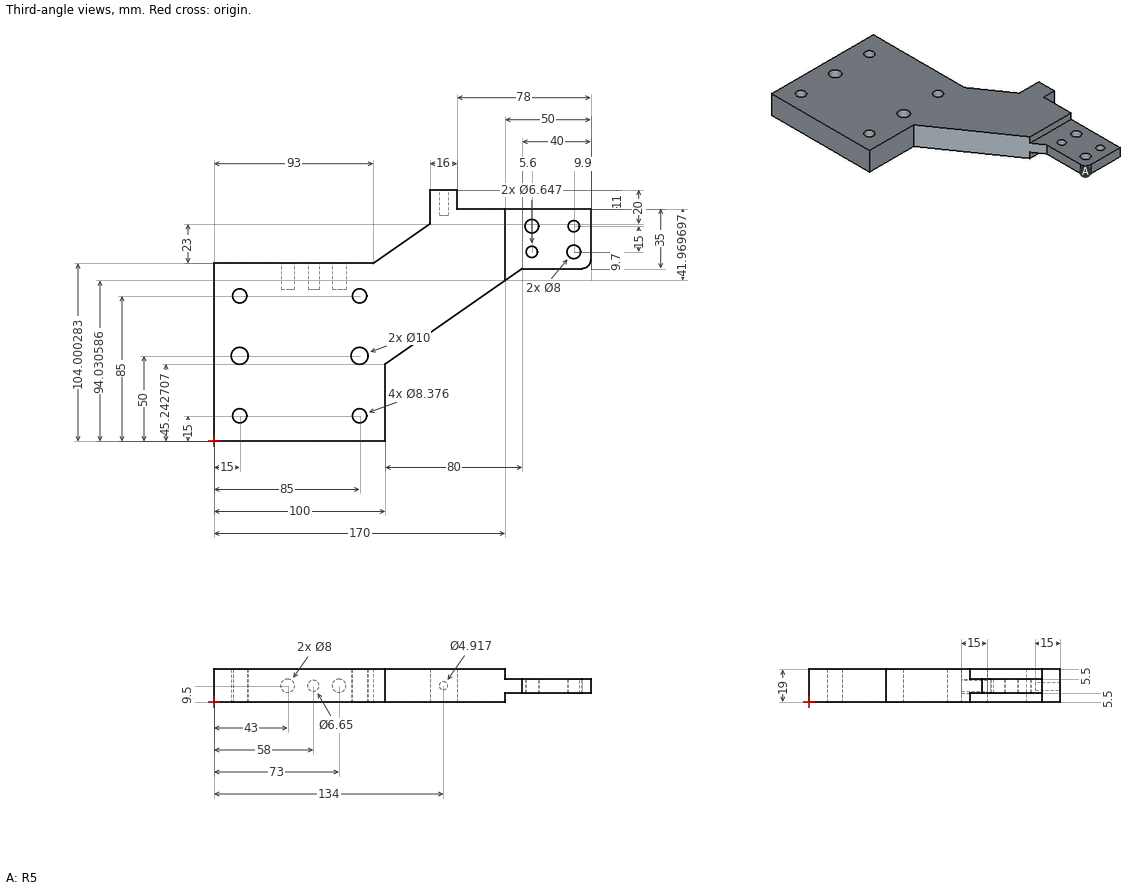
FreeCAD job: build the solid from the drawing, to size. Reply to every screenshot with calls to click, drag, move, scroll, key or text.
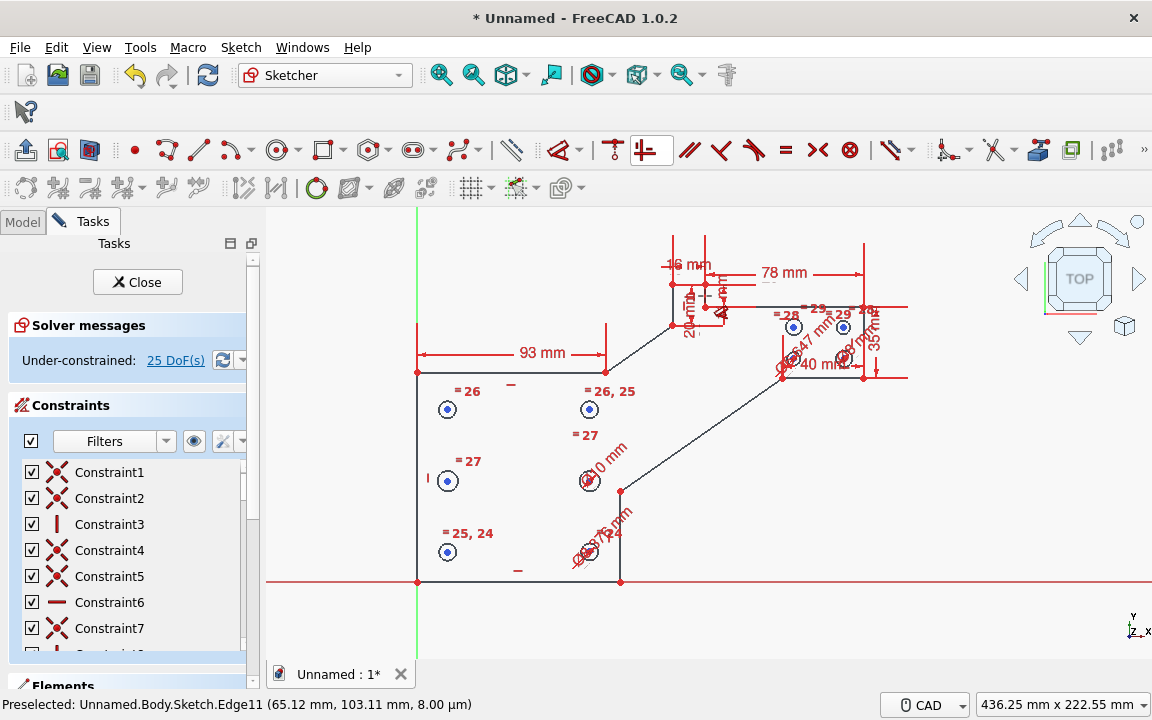
click(590, 552)
click(503, 616)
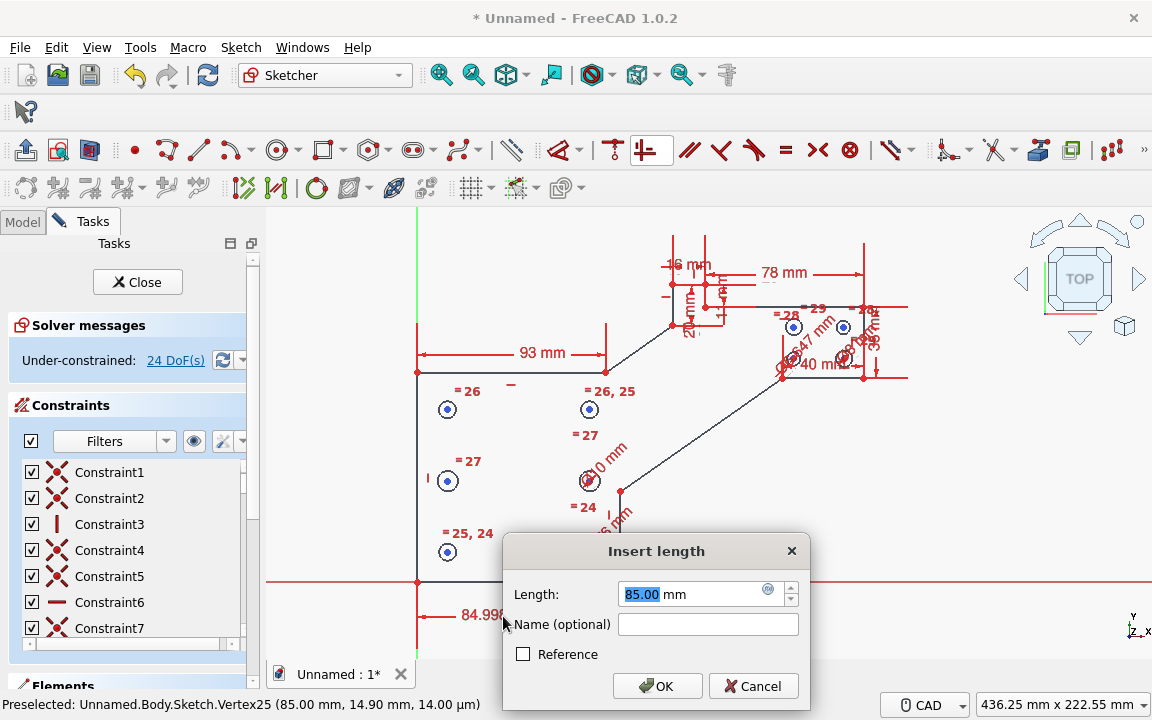
text(85)
key(Return)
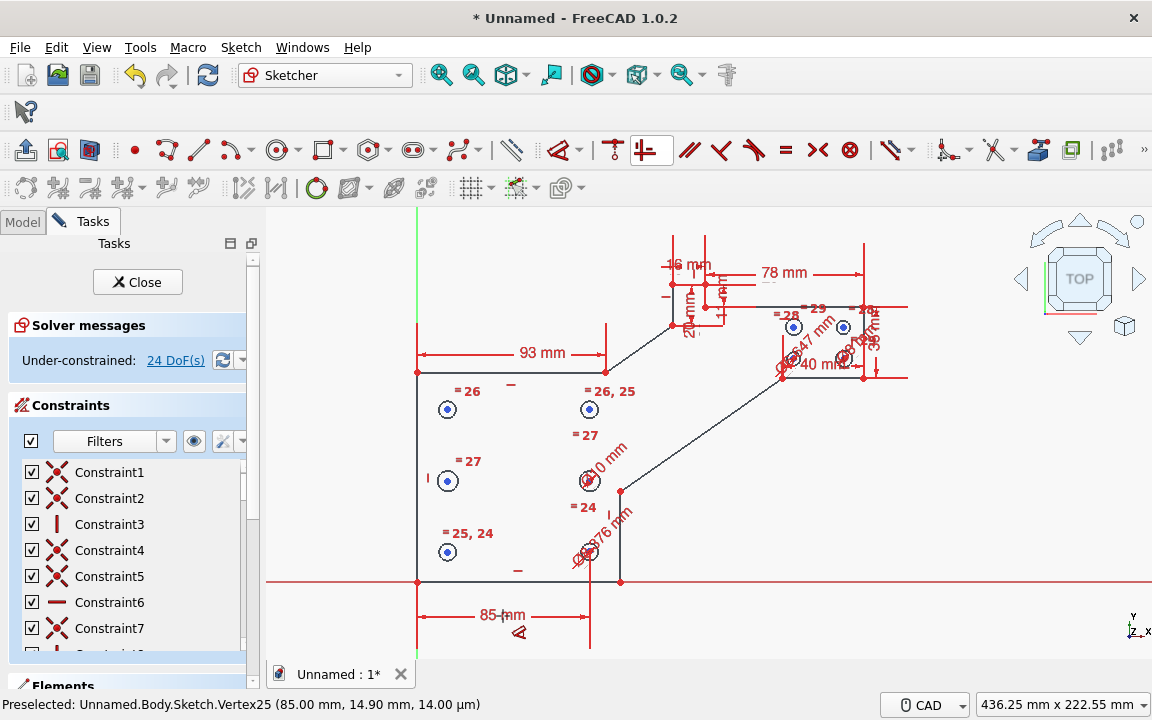
scroll(590, 552, up, 2)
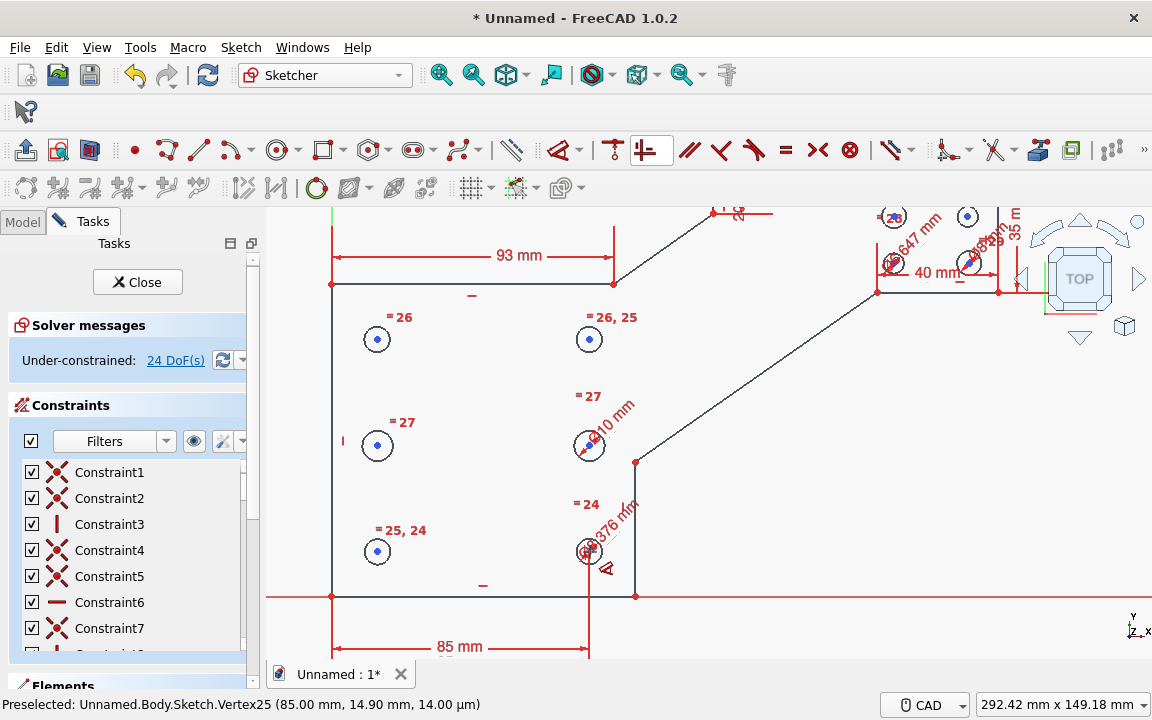
click(589, 552)
click(298, 574)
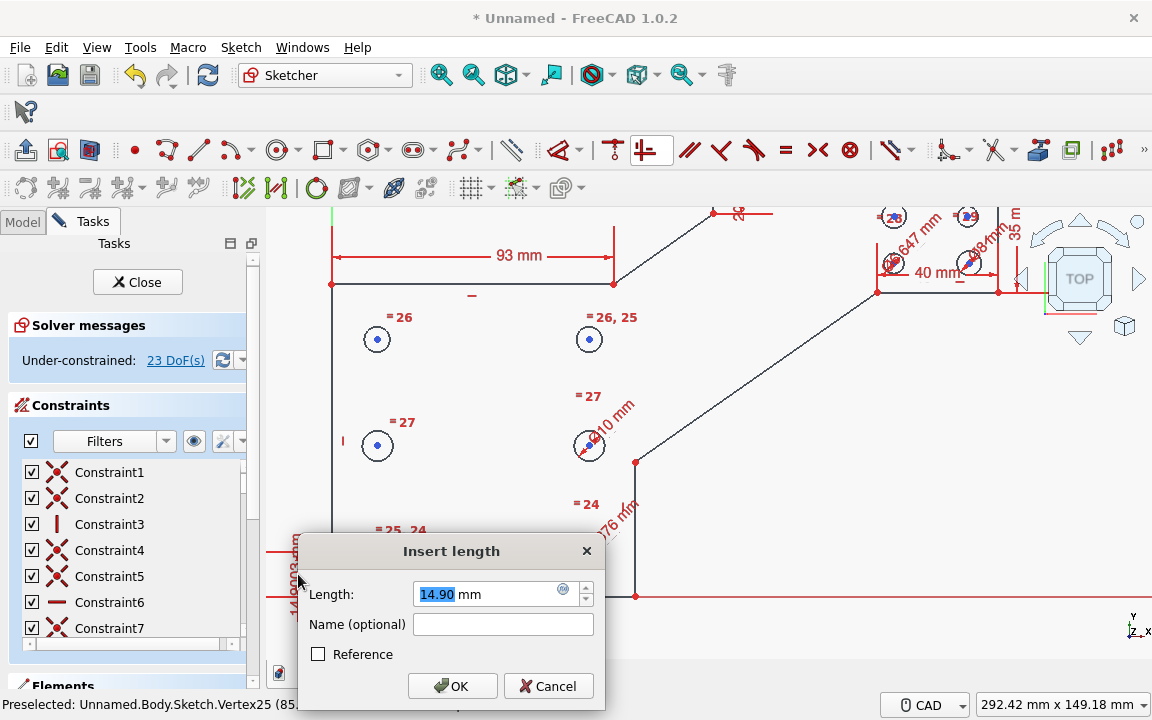
text(15)
key(Return)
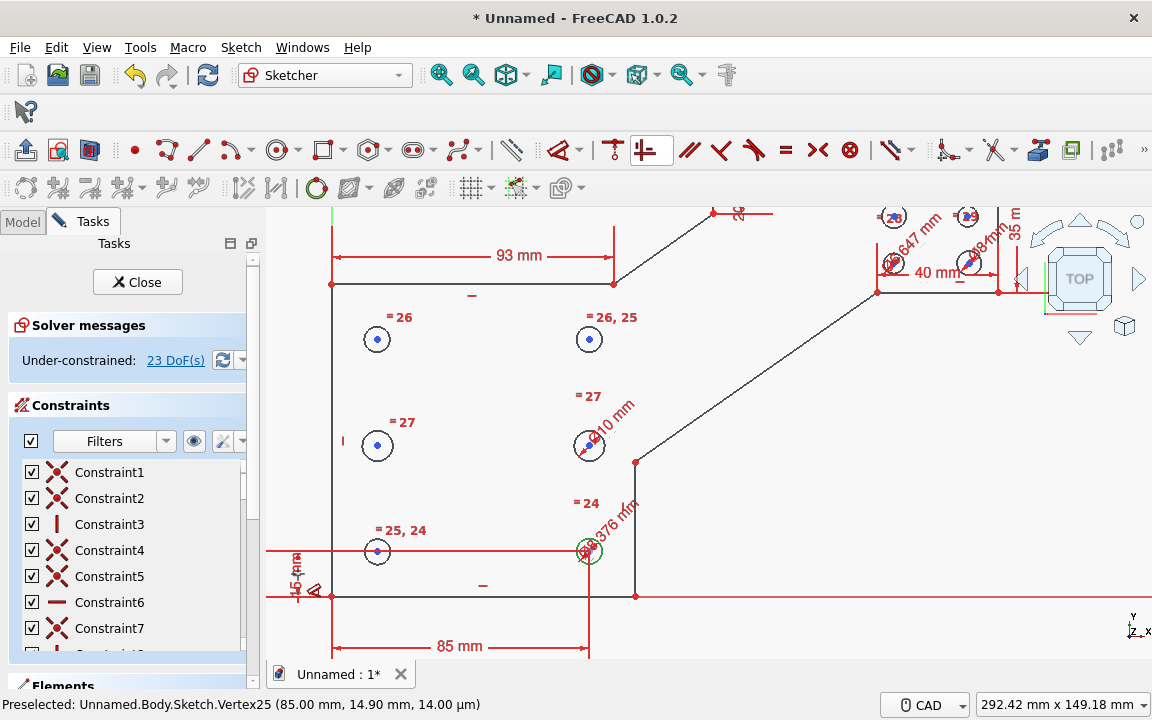
click(378, 552)
click(355, 631)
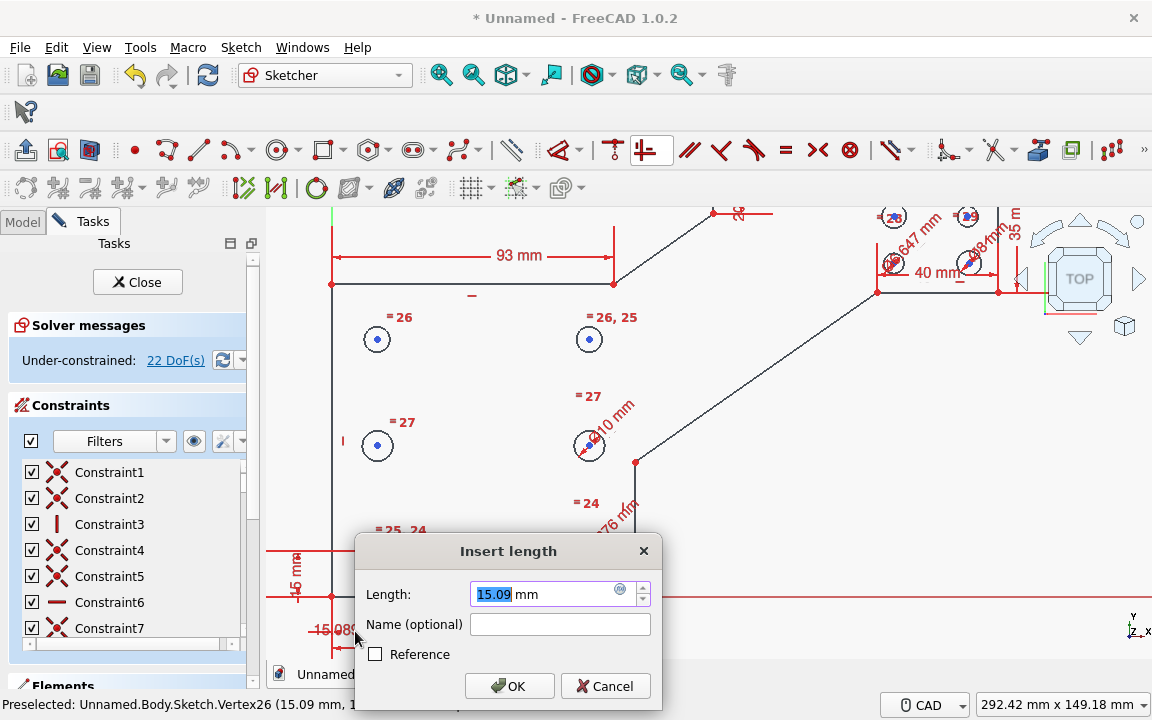
text(15)
key(Return)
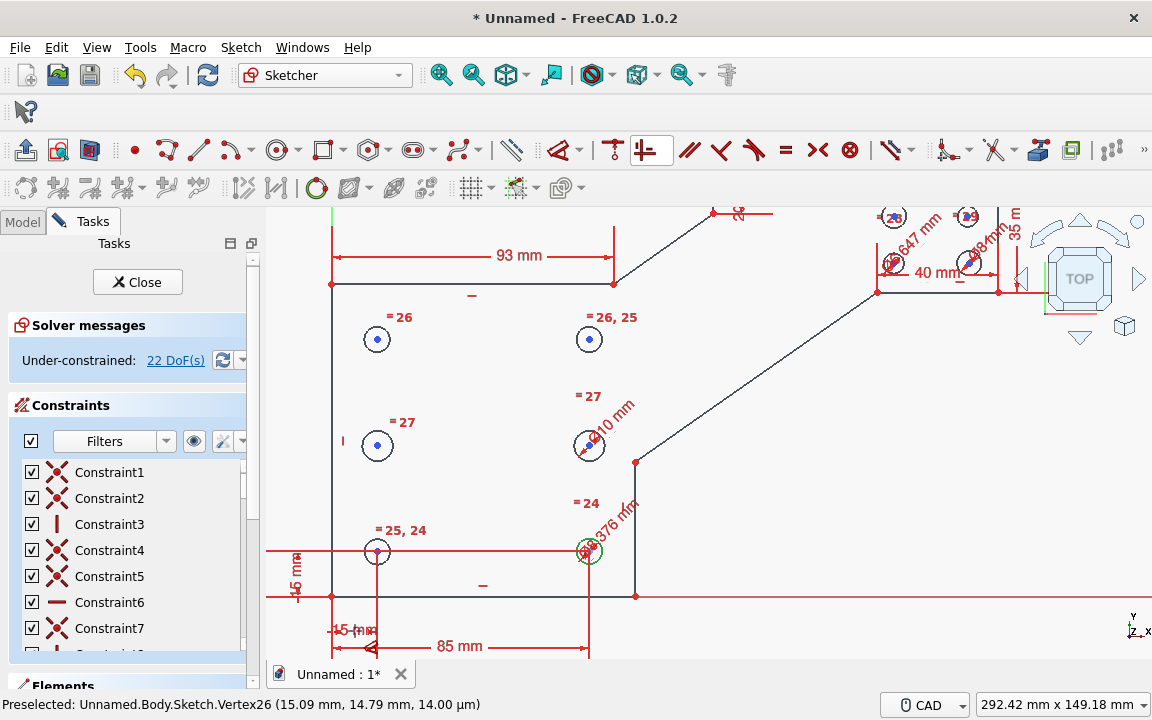
click(377, 552)
click(411, 574)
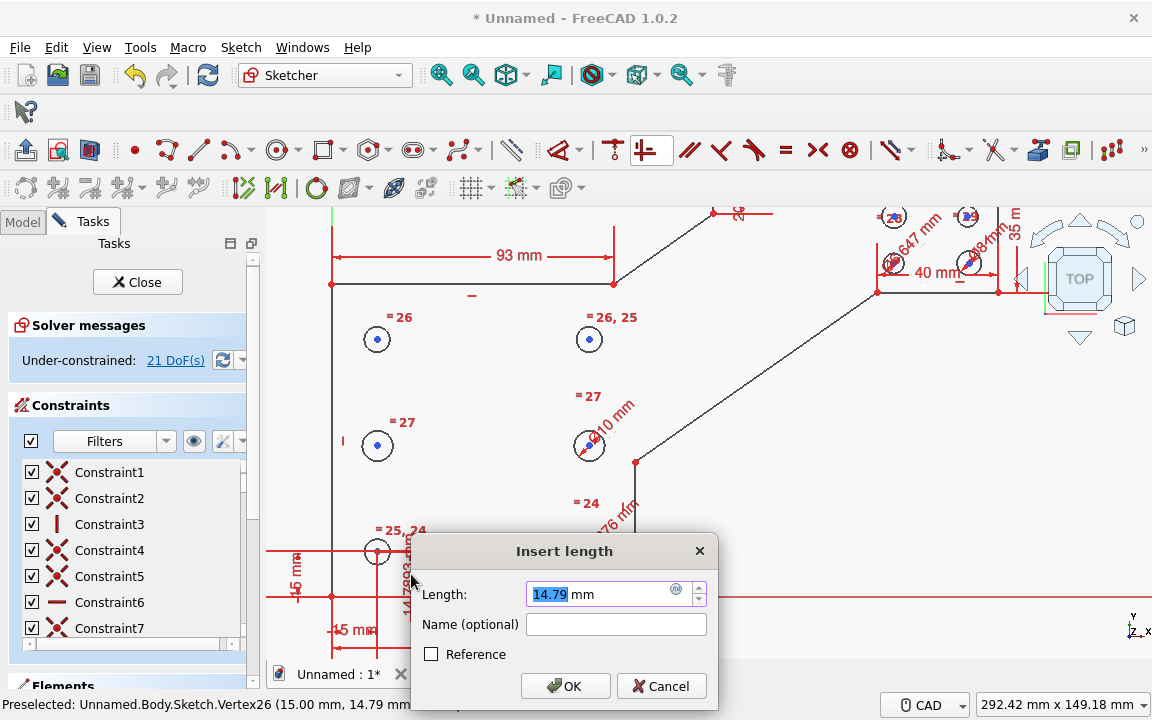
text(15)
key(Return)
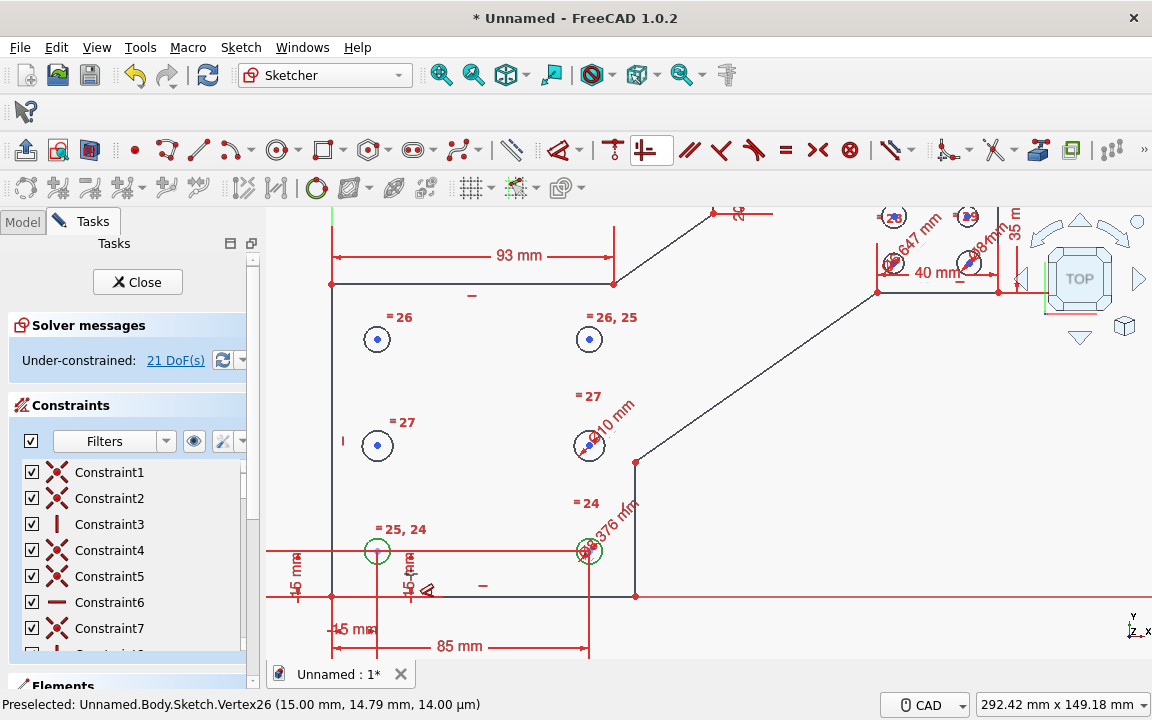
click(589, 446)
click(551, 631)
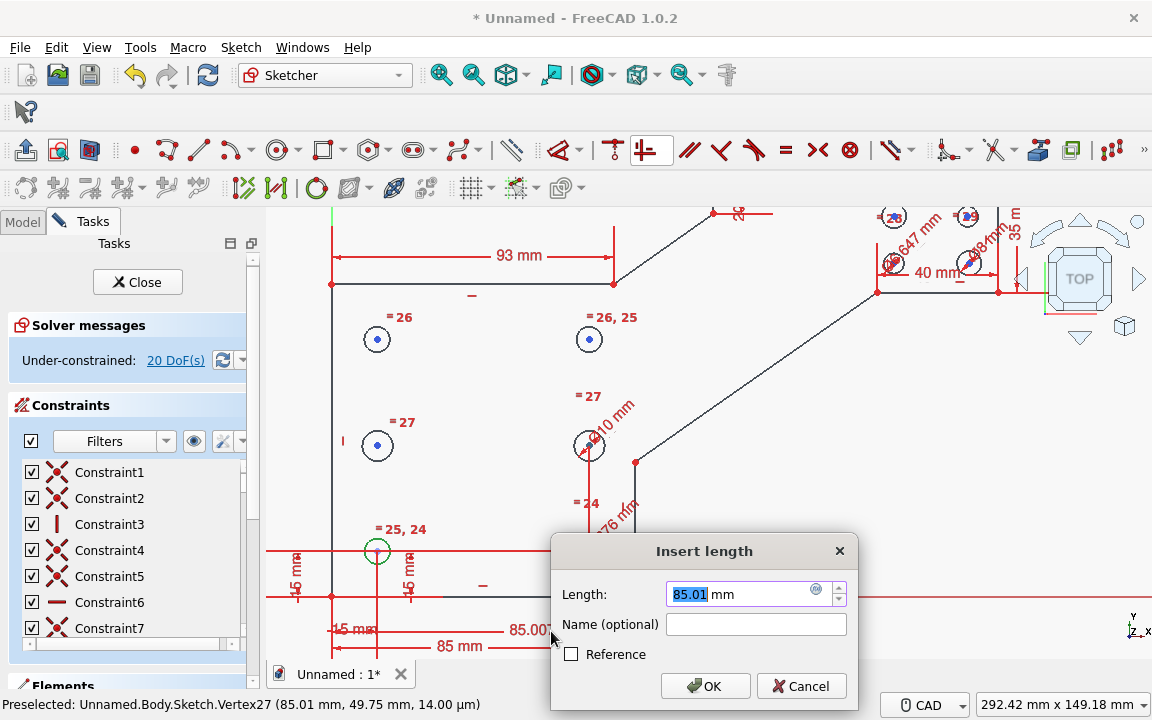
text(85)
key(Return)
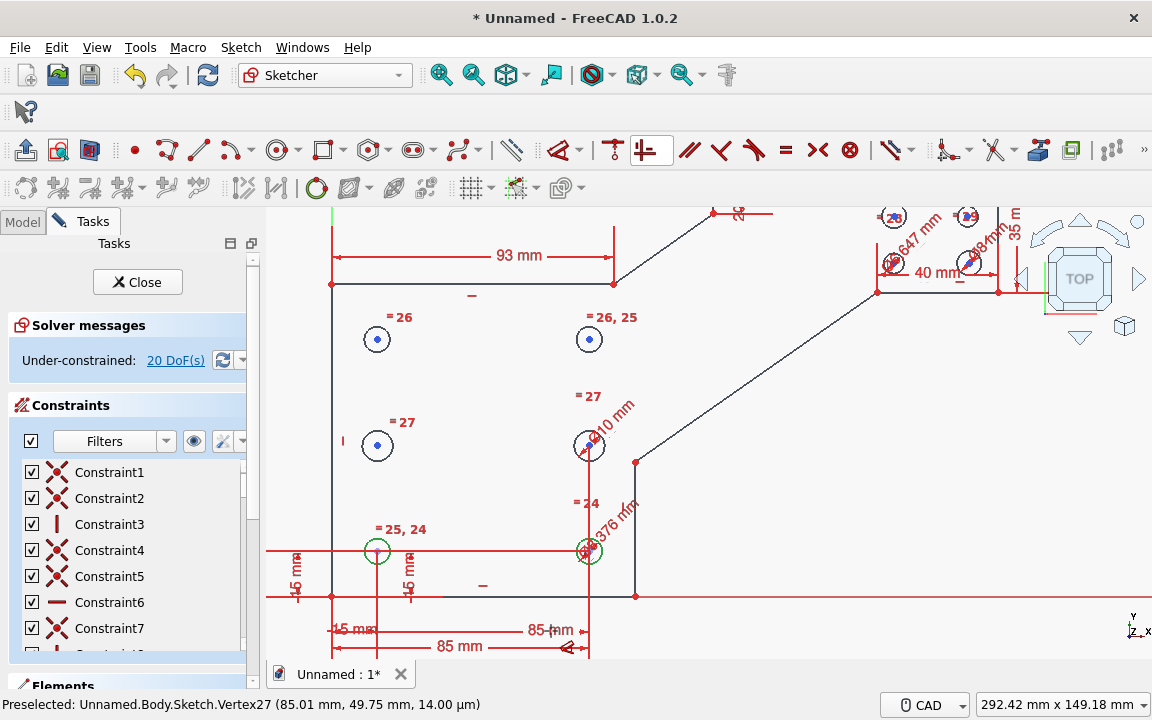
click(589, 446)
click(298, 521)